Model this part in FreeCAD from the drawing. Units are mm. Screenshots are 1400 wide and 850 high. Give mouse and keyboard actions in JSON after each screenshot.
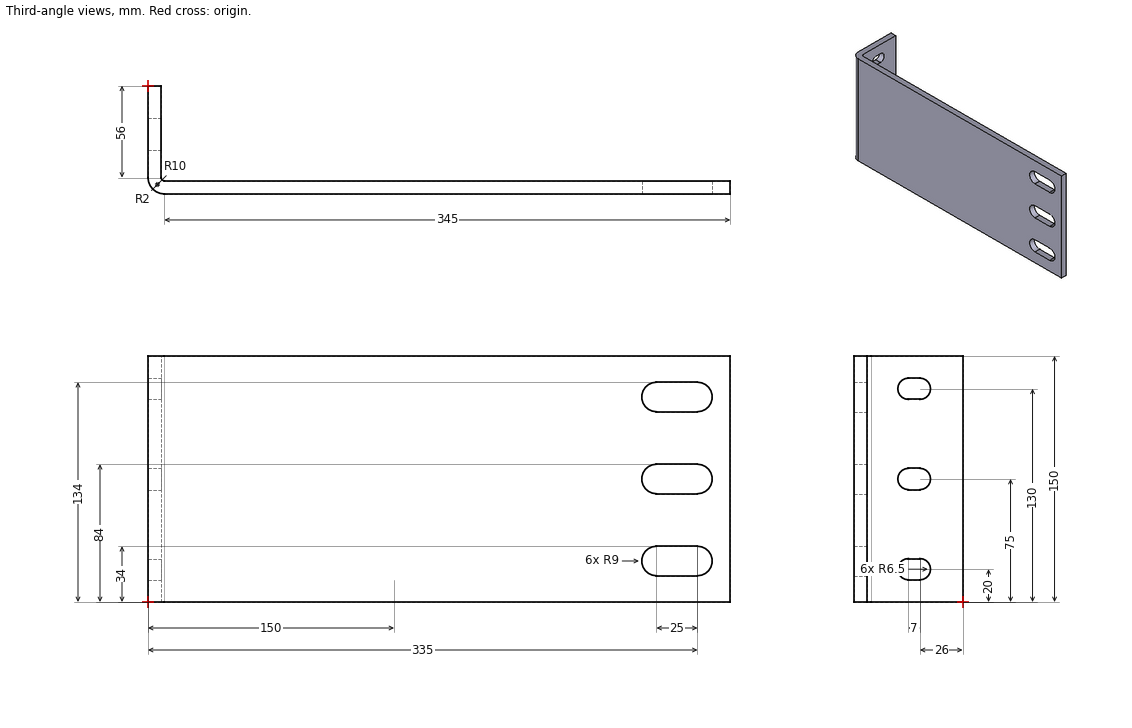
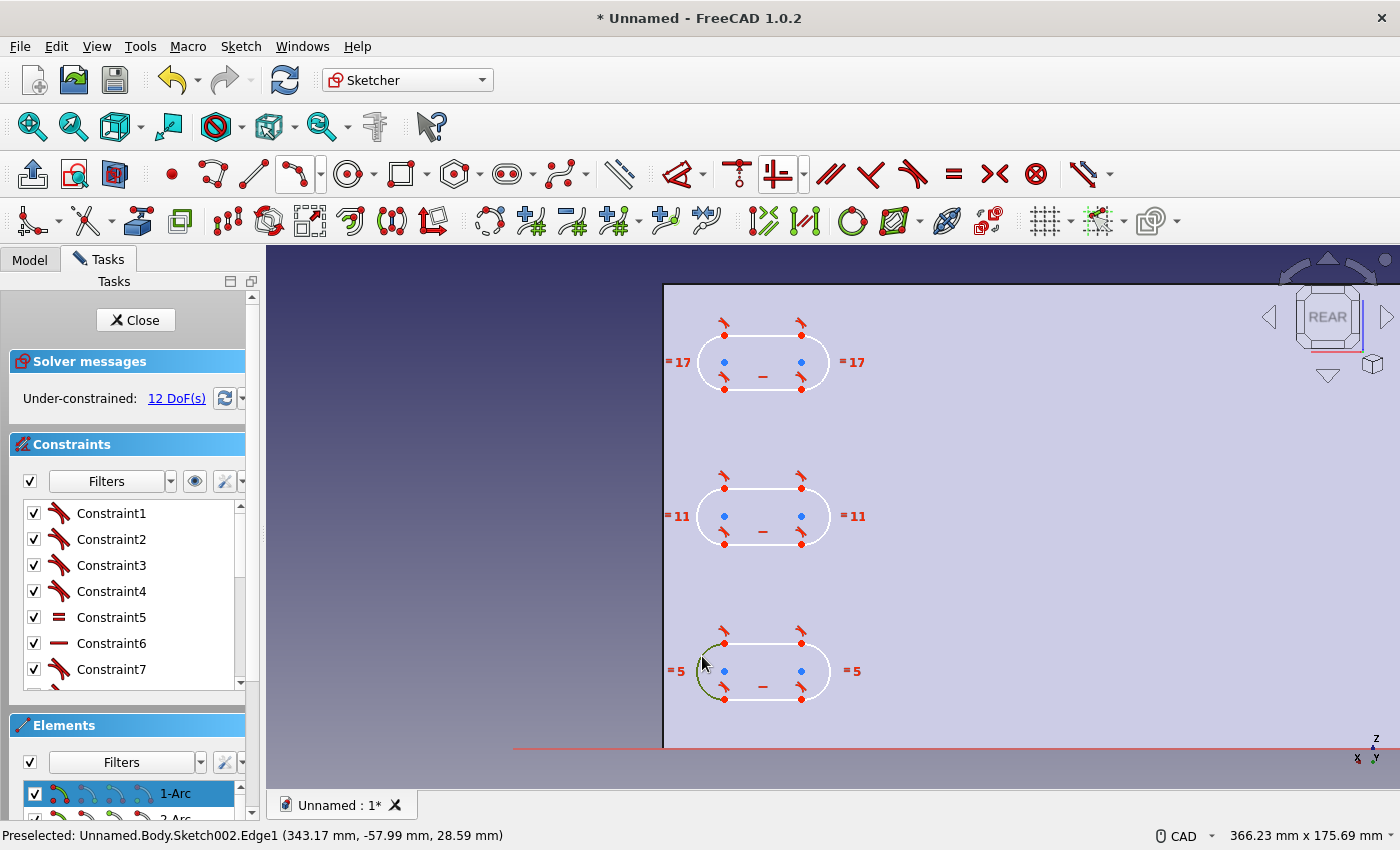
{"action": "left_click", "coordinate": [702, 501]}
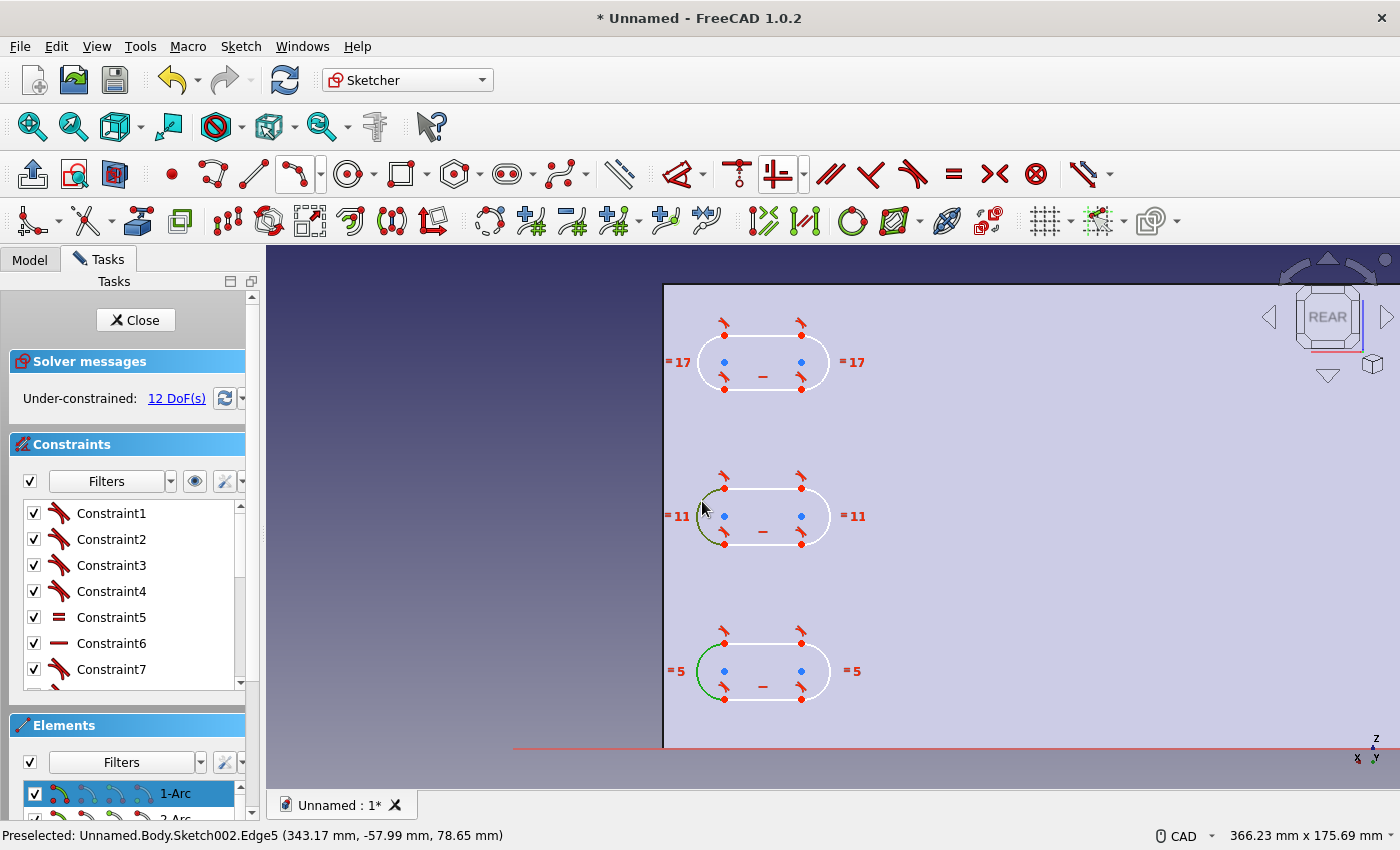
{"action": "left_click", "coordinate": [703, 347]}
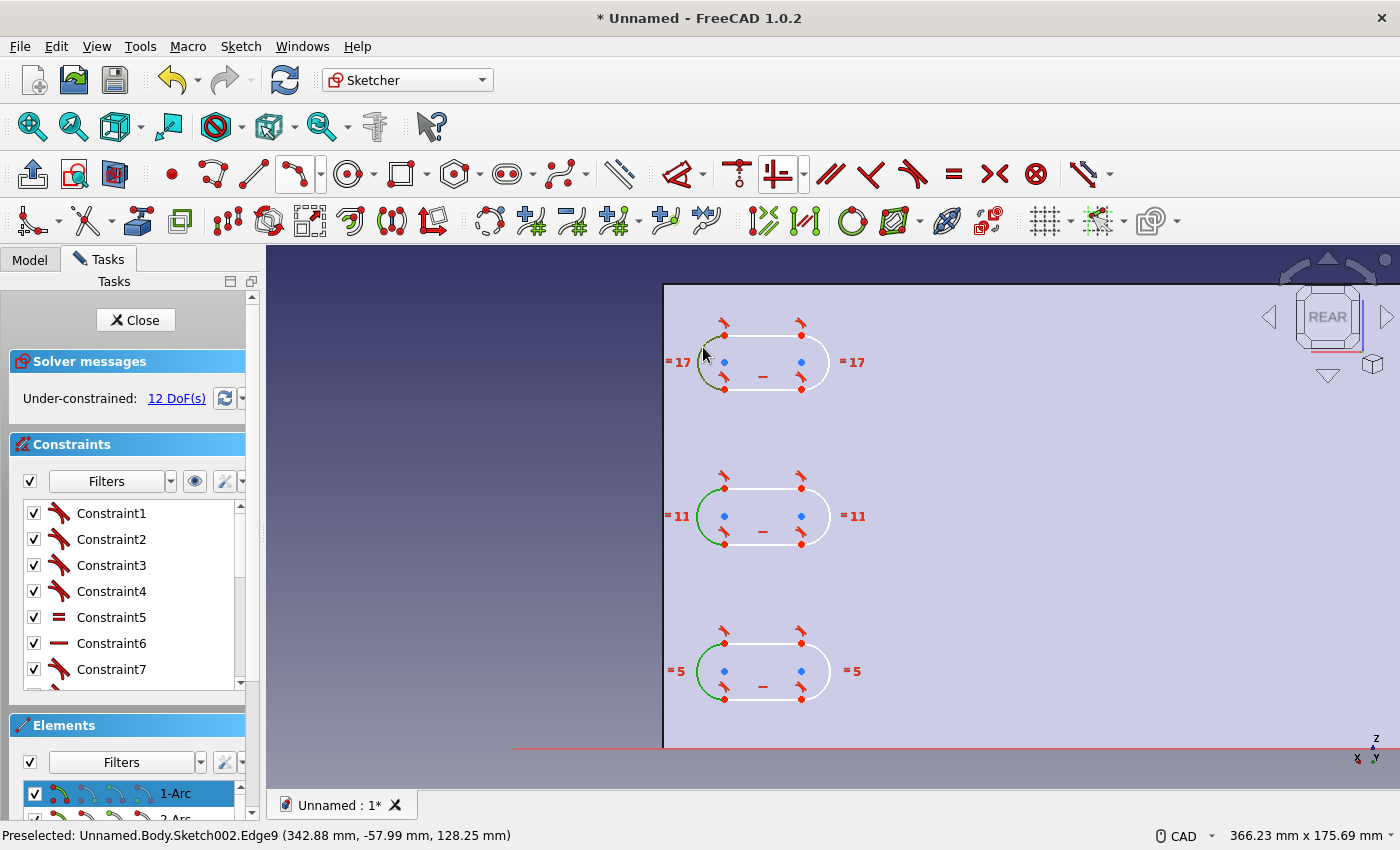
{"action": "left_click", "coordinate": [954, 174]}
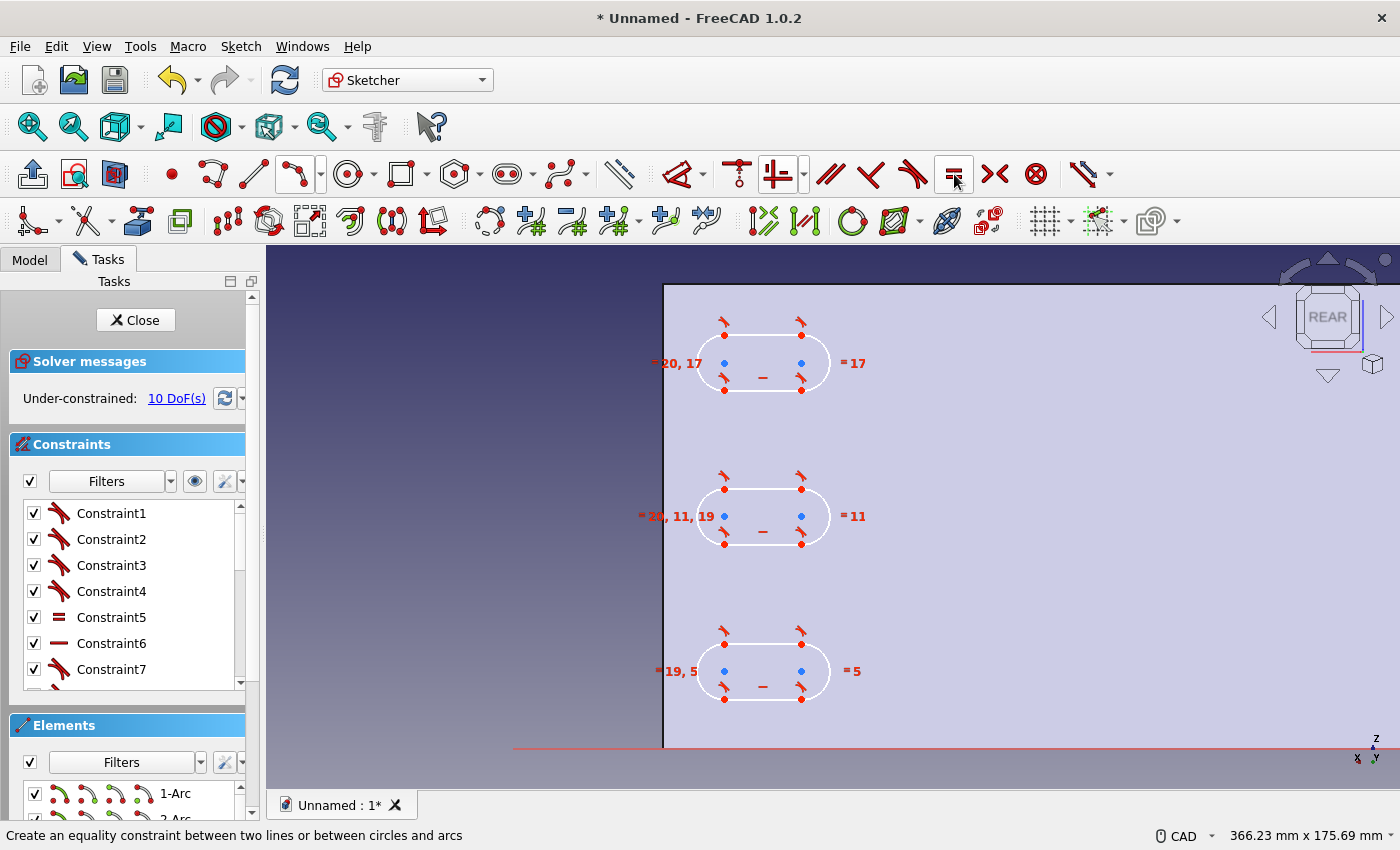
{"action": "left_click", "coordinate": [676, 174]}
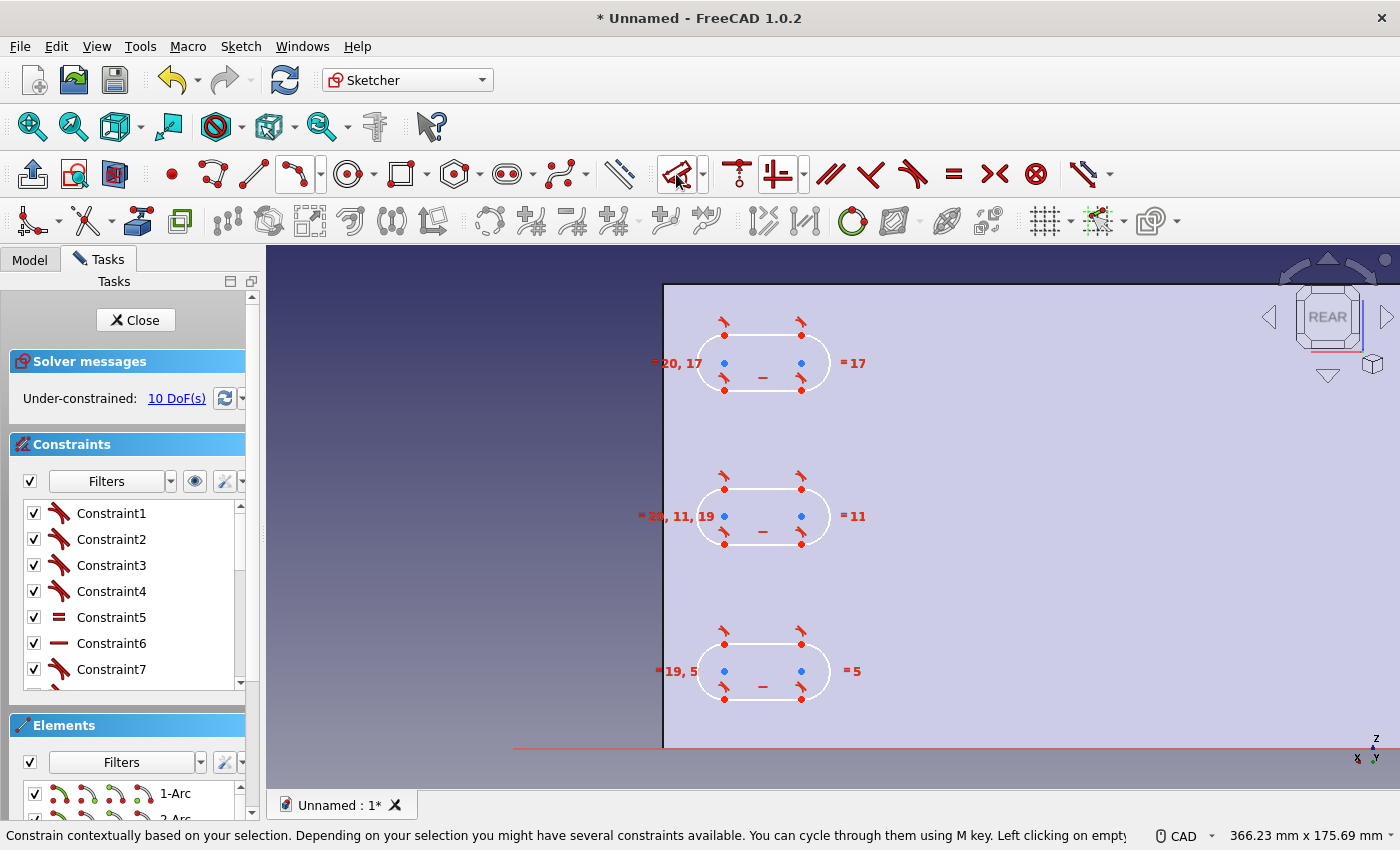
{"action": "scroll", "coordinate": [702, 656], "scroll_direction": "up", "scroll_amount": 2}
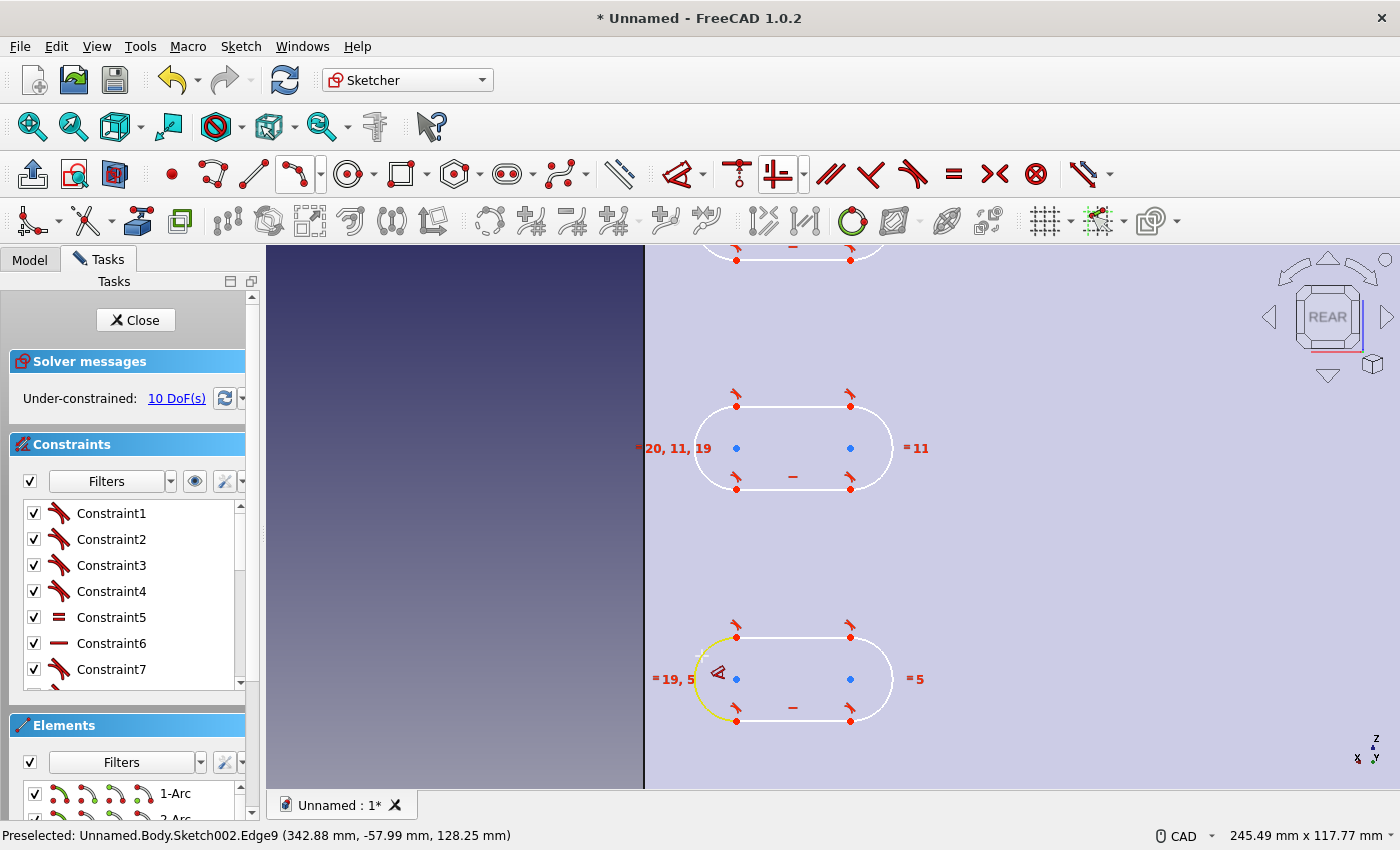
{"action": "left_click", "coordinate": [702, 655]}
{"action": "left_click", "coordinate": [676, 636]}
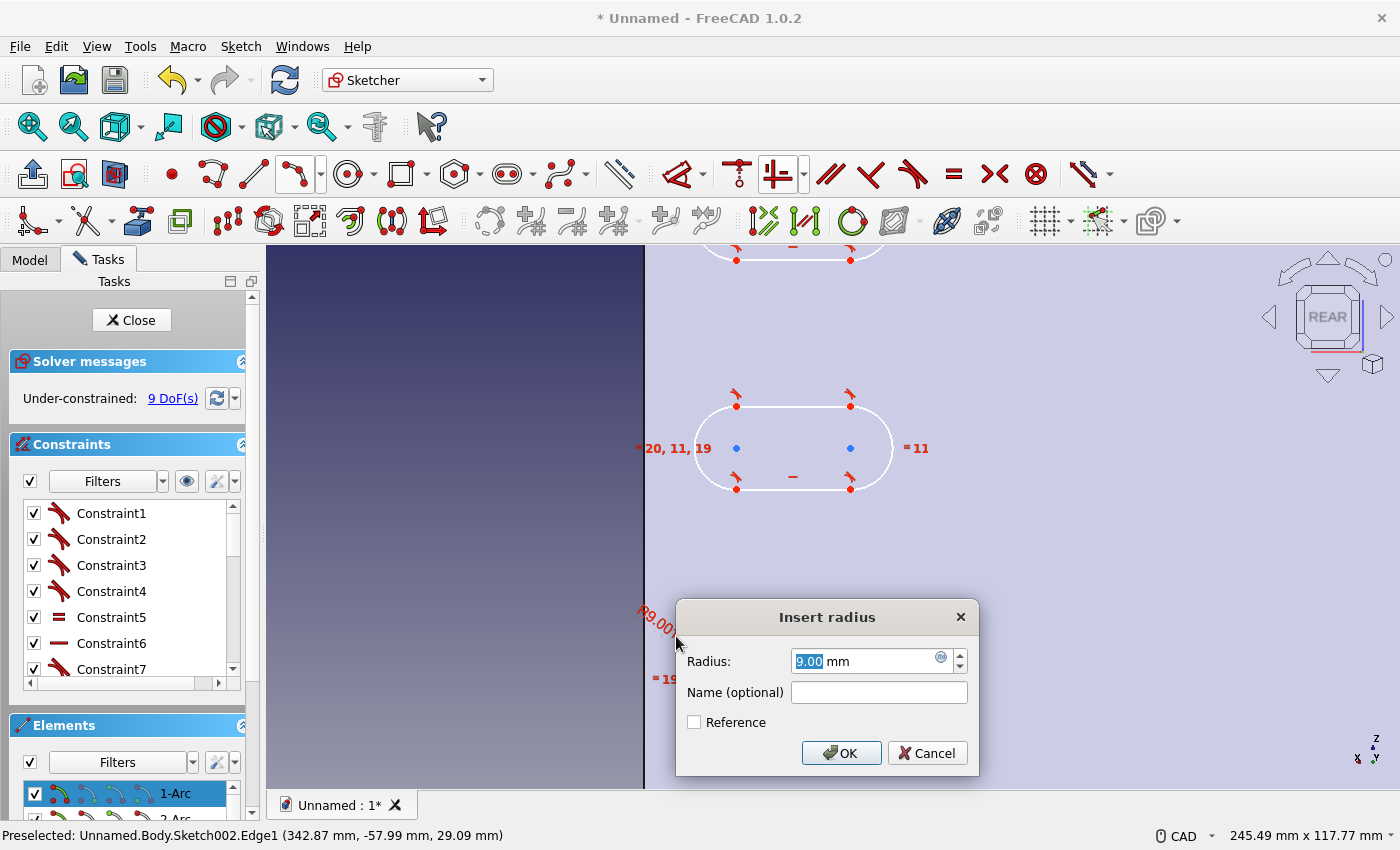
{"action": "type", "text": "9"}
{"action": "key", "text": "Return"}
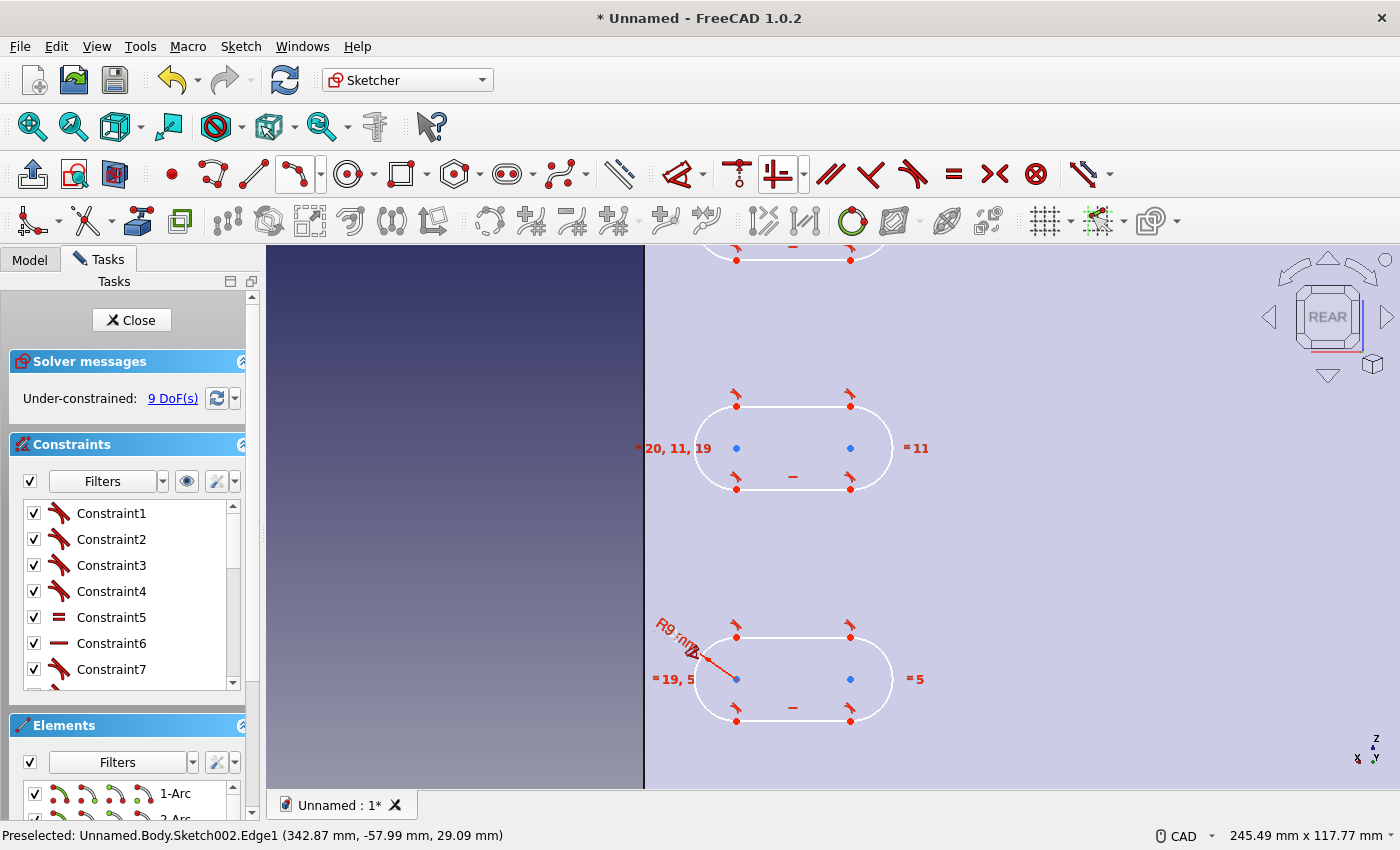
{"action": "left_click", "coordinate": [771, 638]}
{"action": "left_click", "coordinate": [794, 672]}